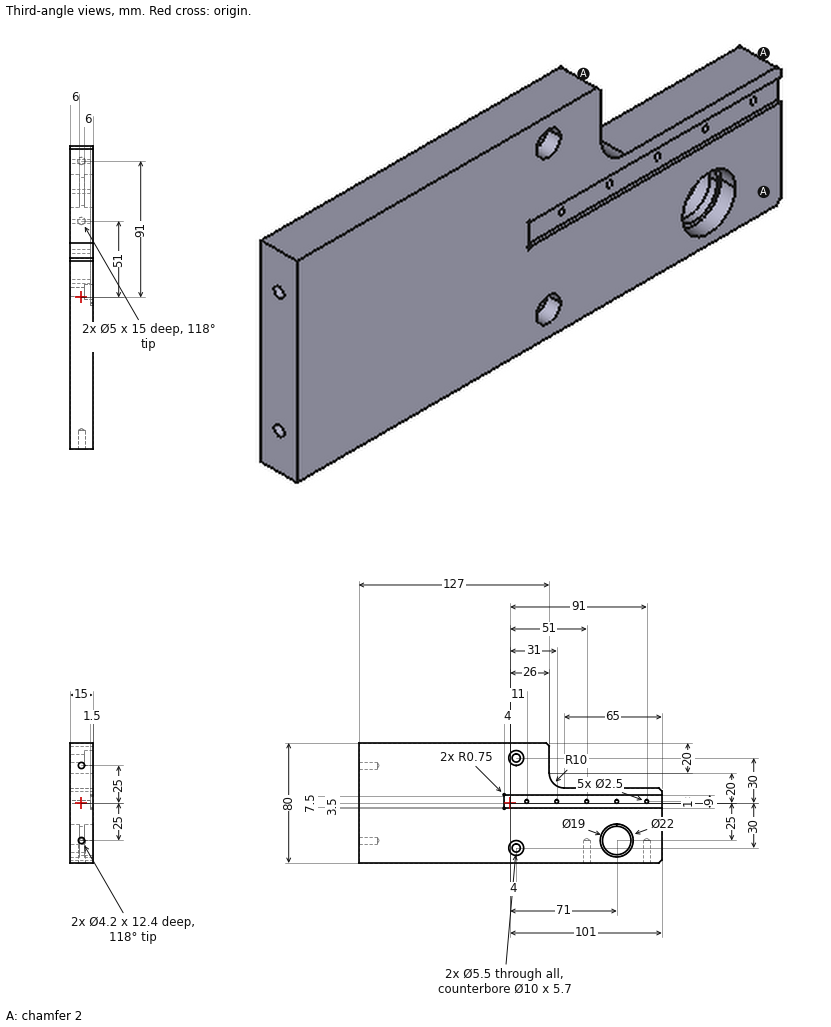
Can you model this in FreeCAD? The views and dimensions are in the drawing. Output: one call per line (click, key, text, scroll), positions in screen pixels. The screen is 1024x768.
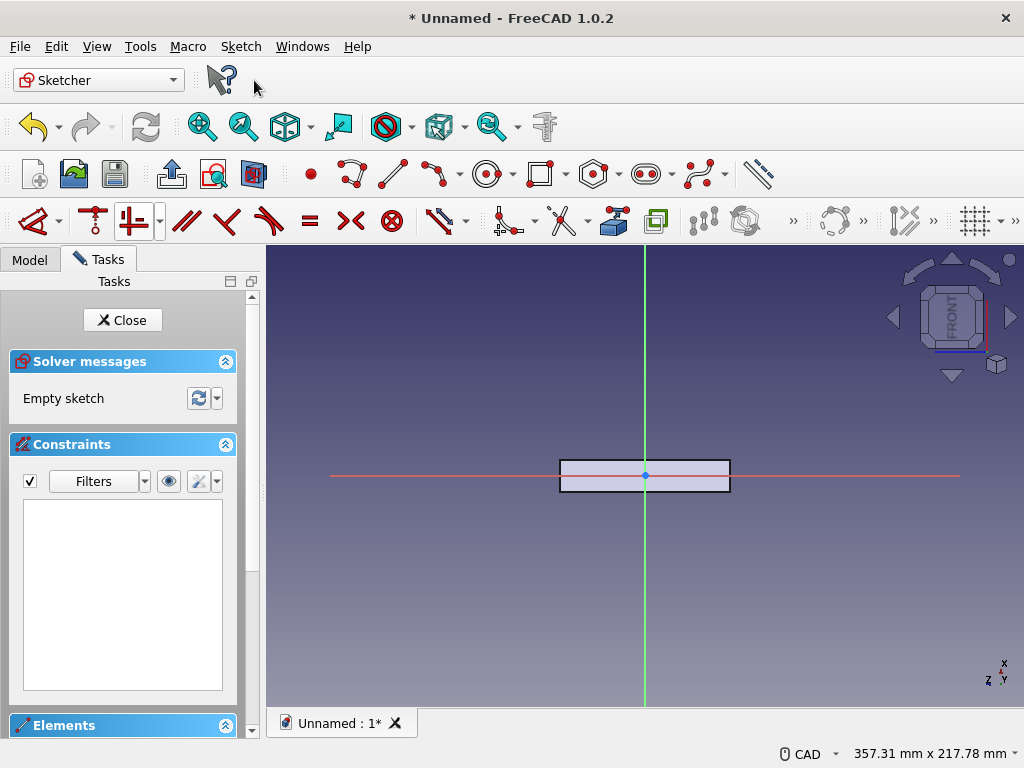
scroll(675, 476, up, 6)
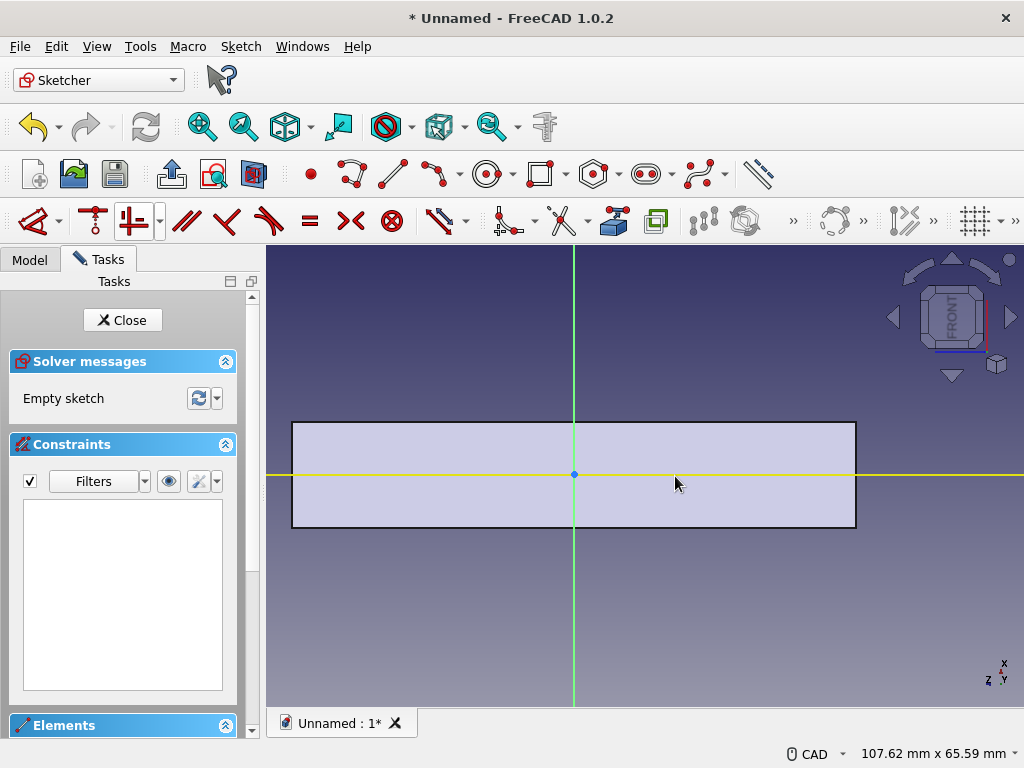
click(486, 174)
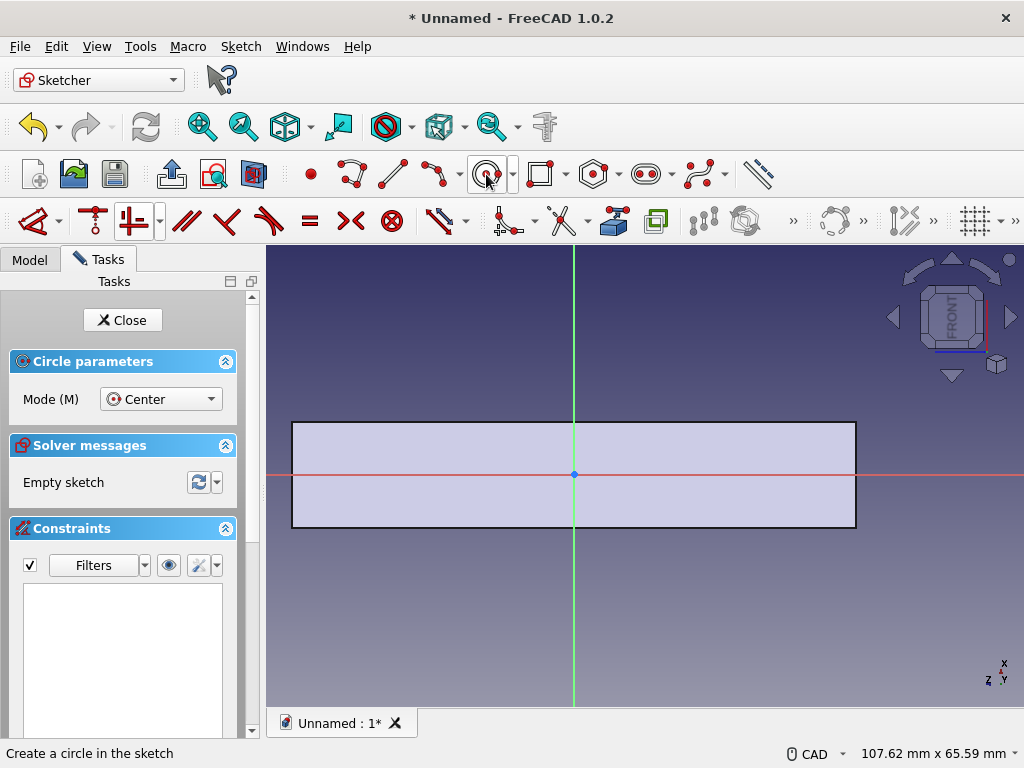
scroll(750, 475, up, 3)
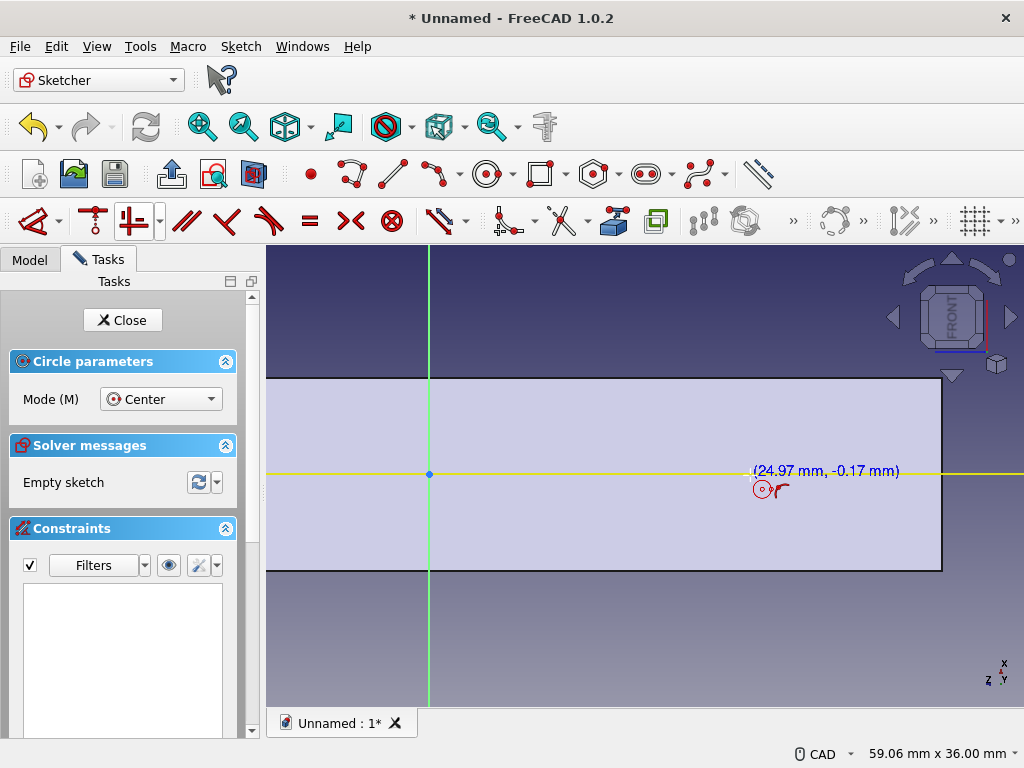
click(750, 474)
click(769, 455)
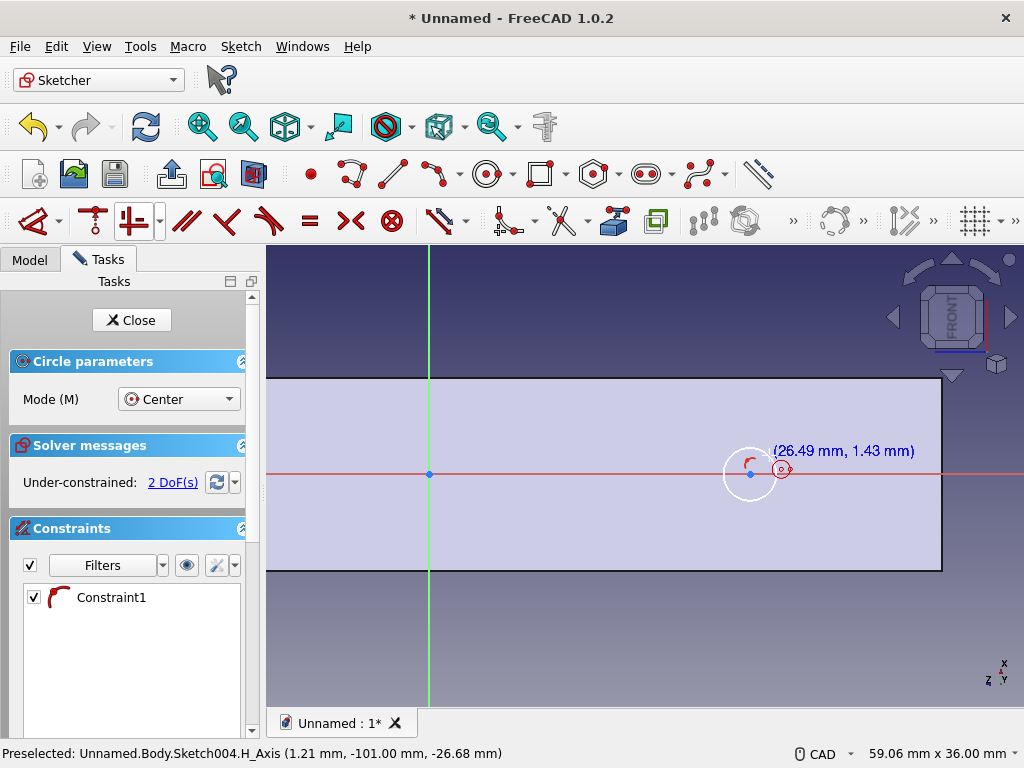
scroll(756, 478, down, 3)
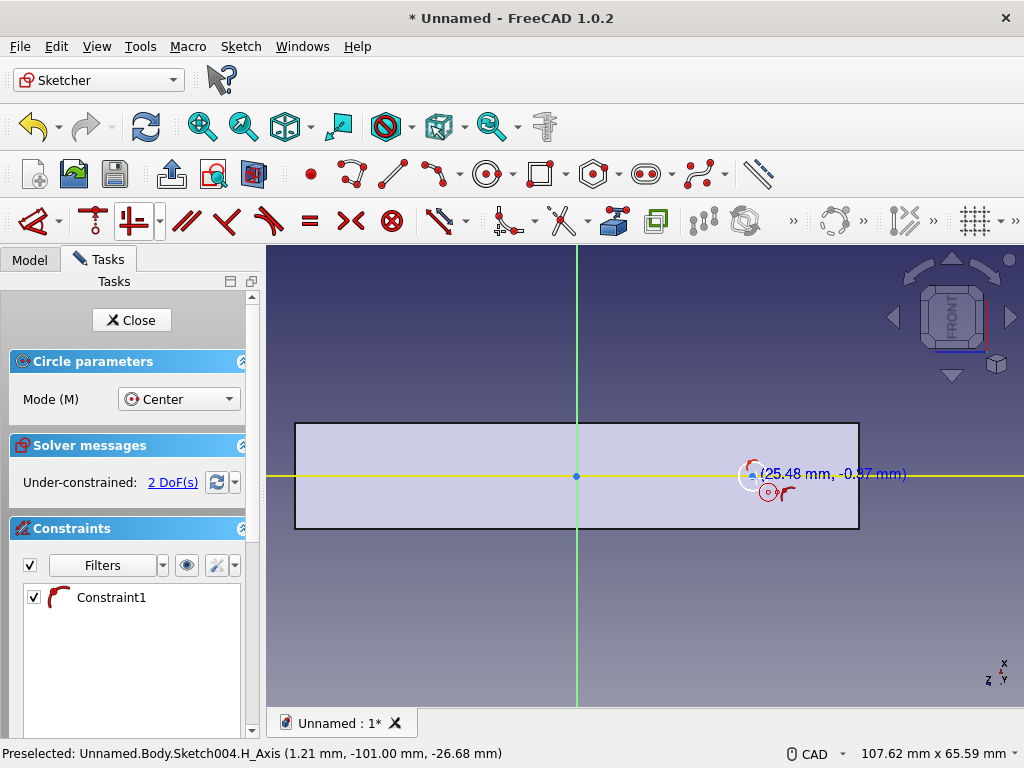
scroll(401, 476, up, 3)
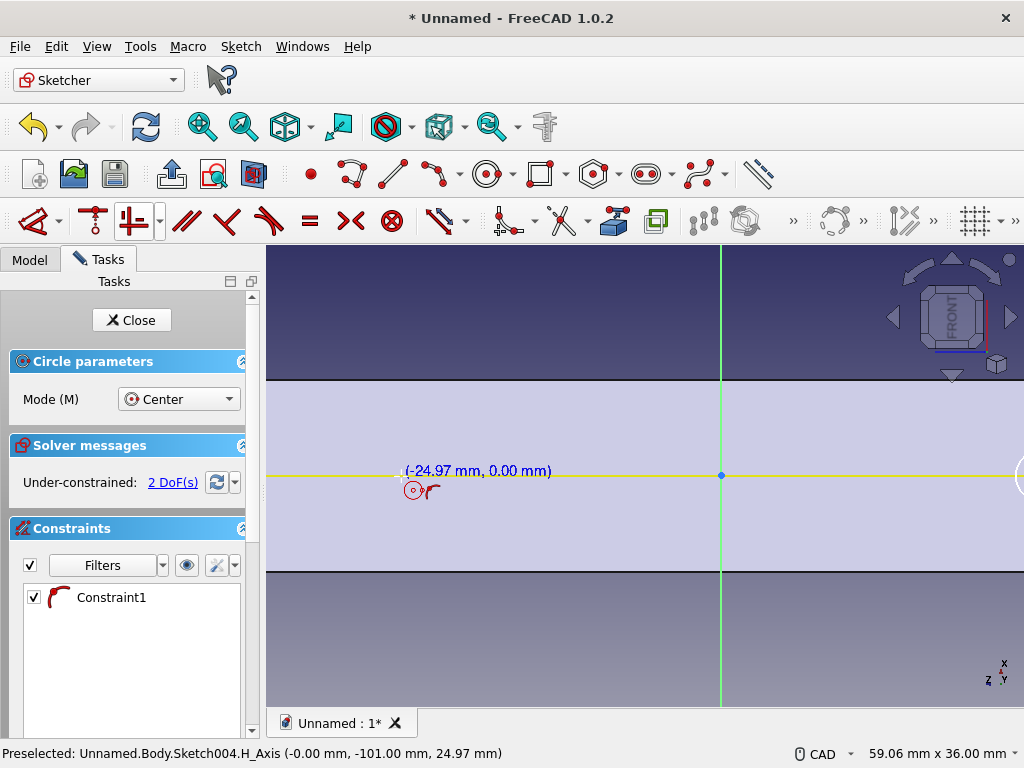
click(400, 476)
click(419, 457)
key(Escape)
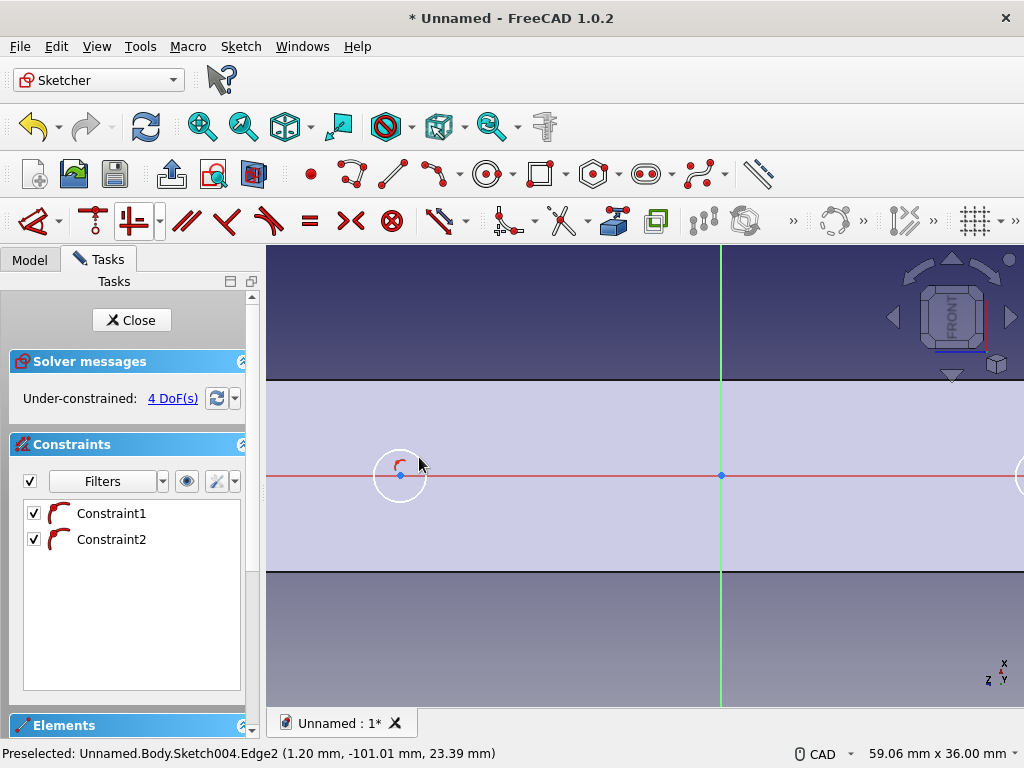
scroll(400, 476, down, 3)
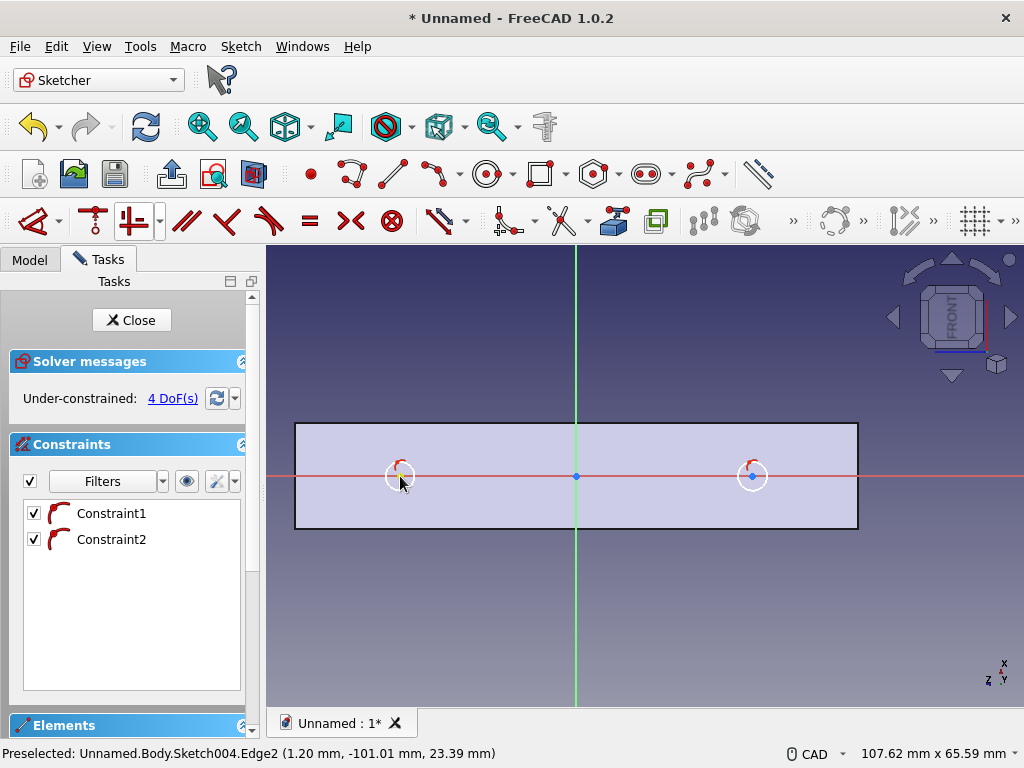
scroll(763, 466, up, 2)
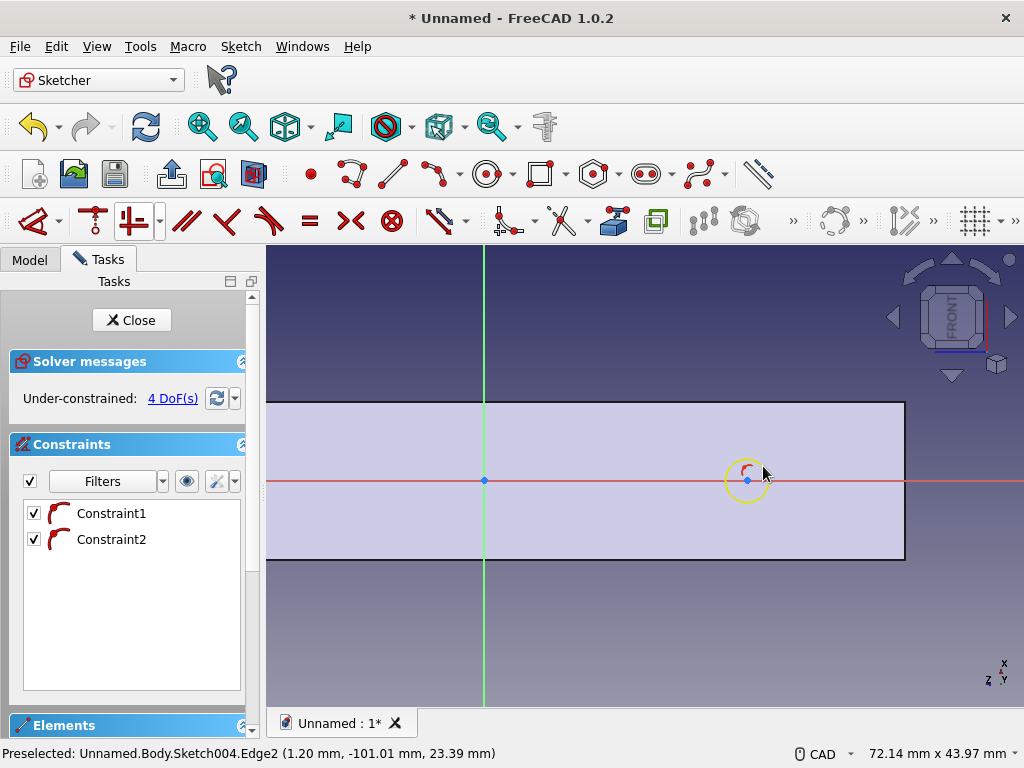
click(762, 466)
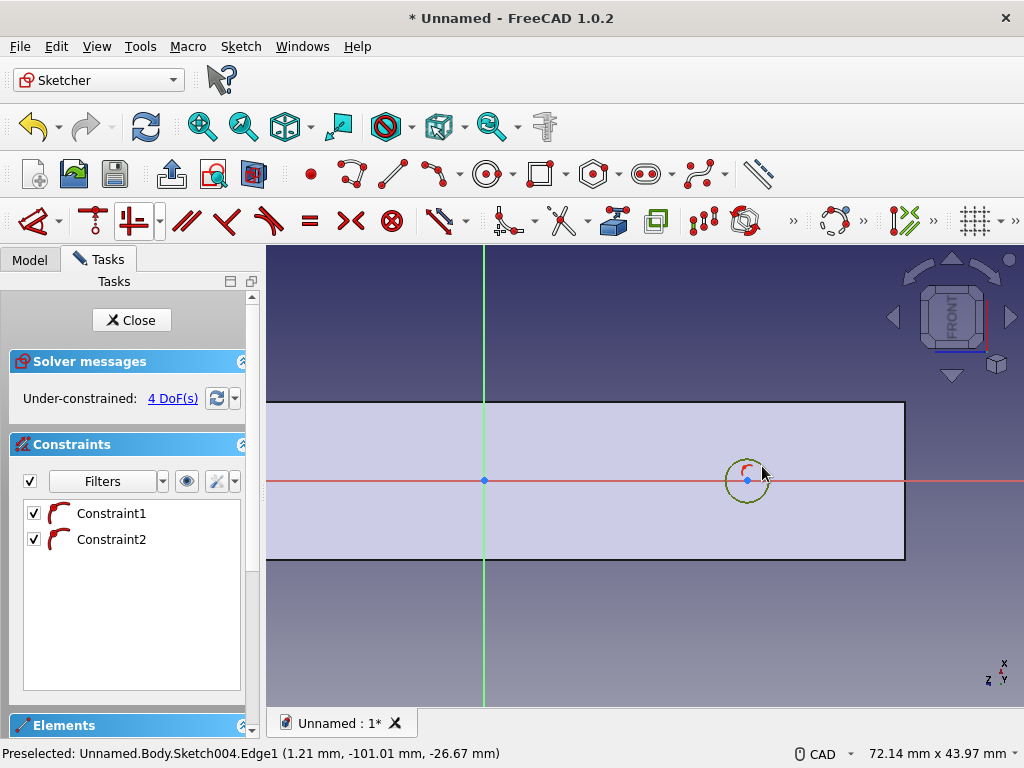
scroll(764, 466, down, 2)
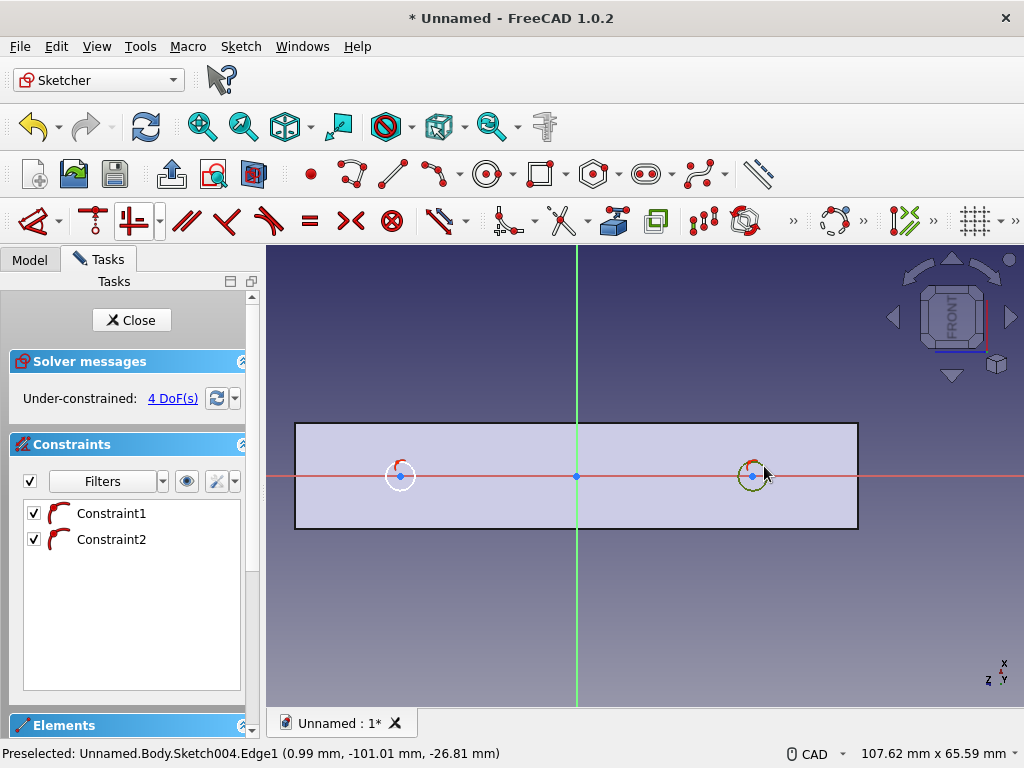
scroll(411, 466, up, 2)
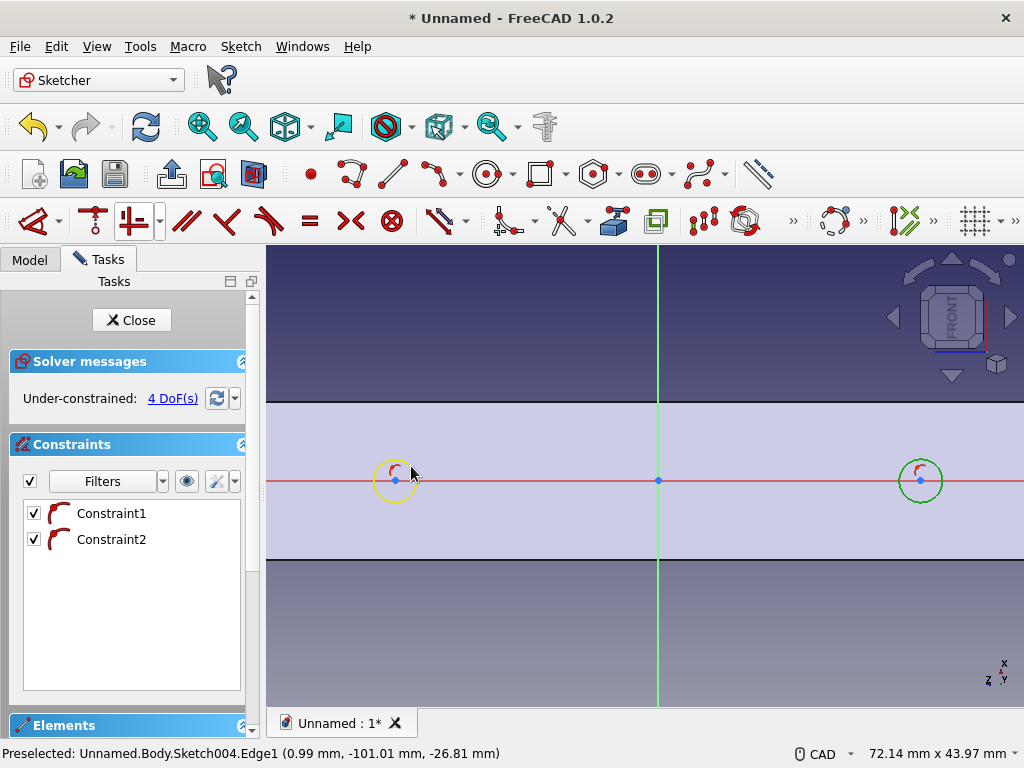
click(410, 466)